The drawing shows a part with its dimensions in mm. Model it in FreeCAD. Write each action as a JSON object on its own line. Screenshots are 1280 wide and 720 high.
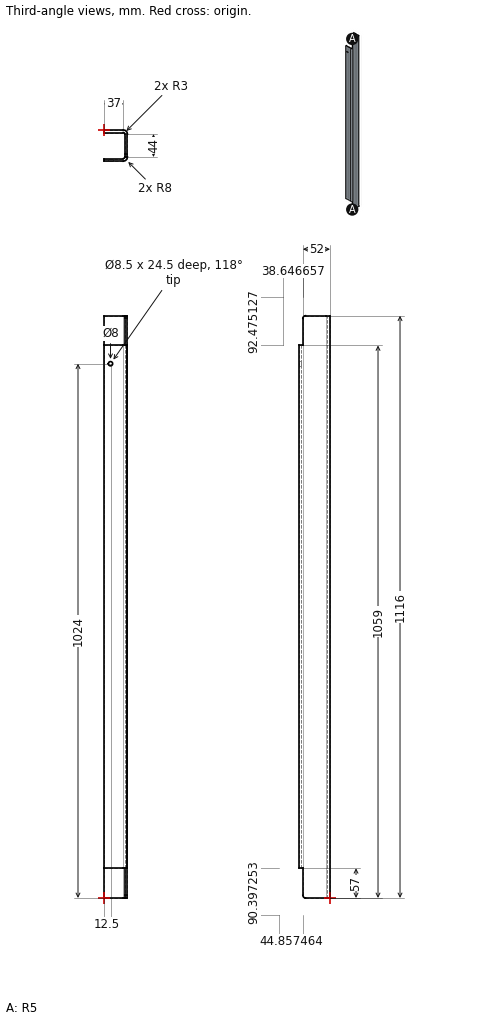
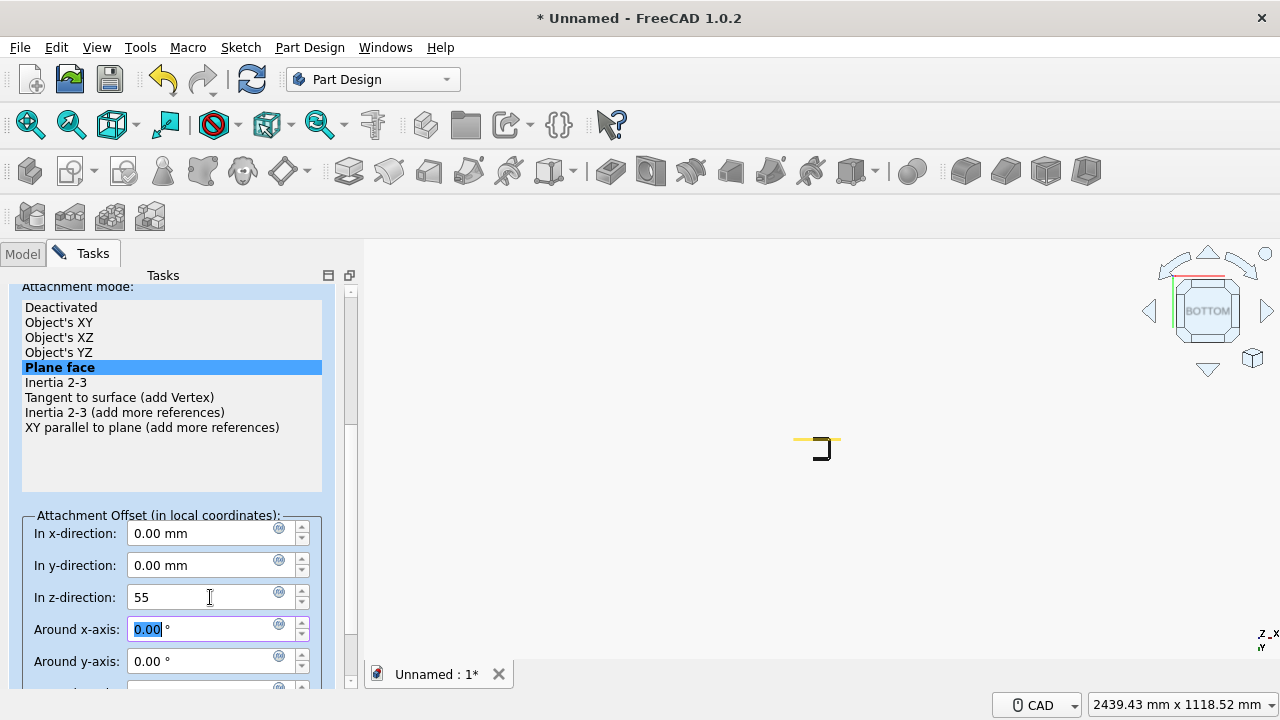
{"action": "scroll", "coordinate": [351, 486], "scroll_direction": "up", "scroll_amount": 5}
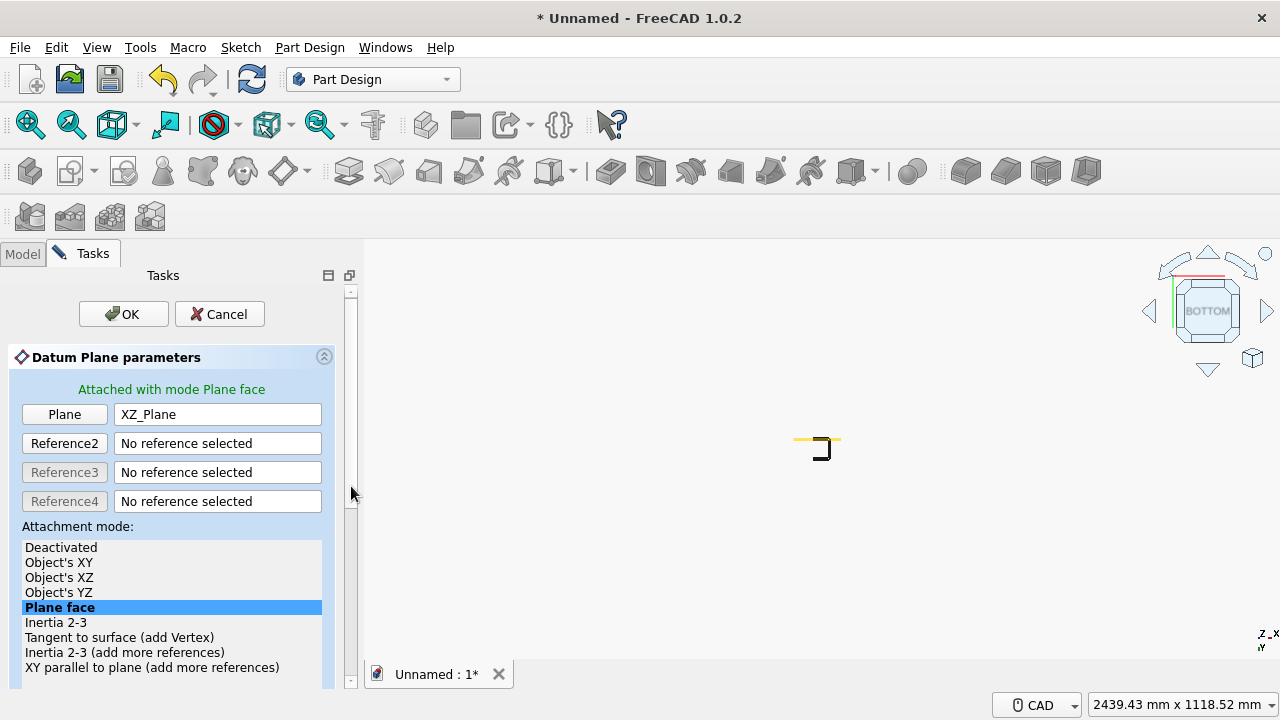
{"action": "left_click", "coordinate": [124, 314]}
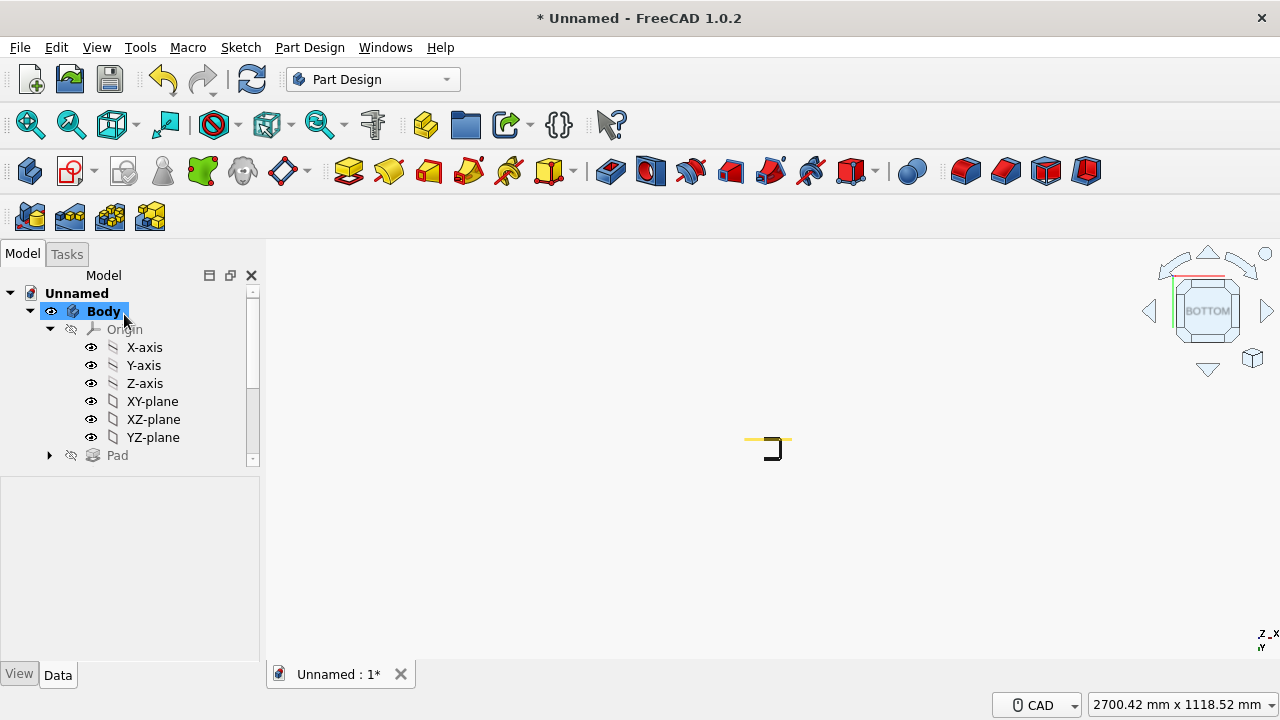
{"action": "scroll", "coordinate": [100, 379], "scroll_direction": "down", "scroll_amount": 3}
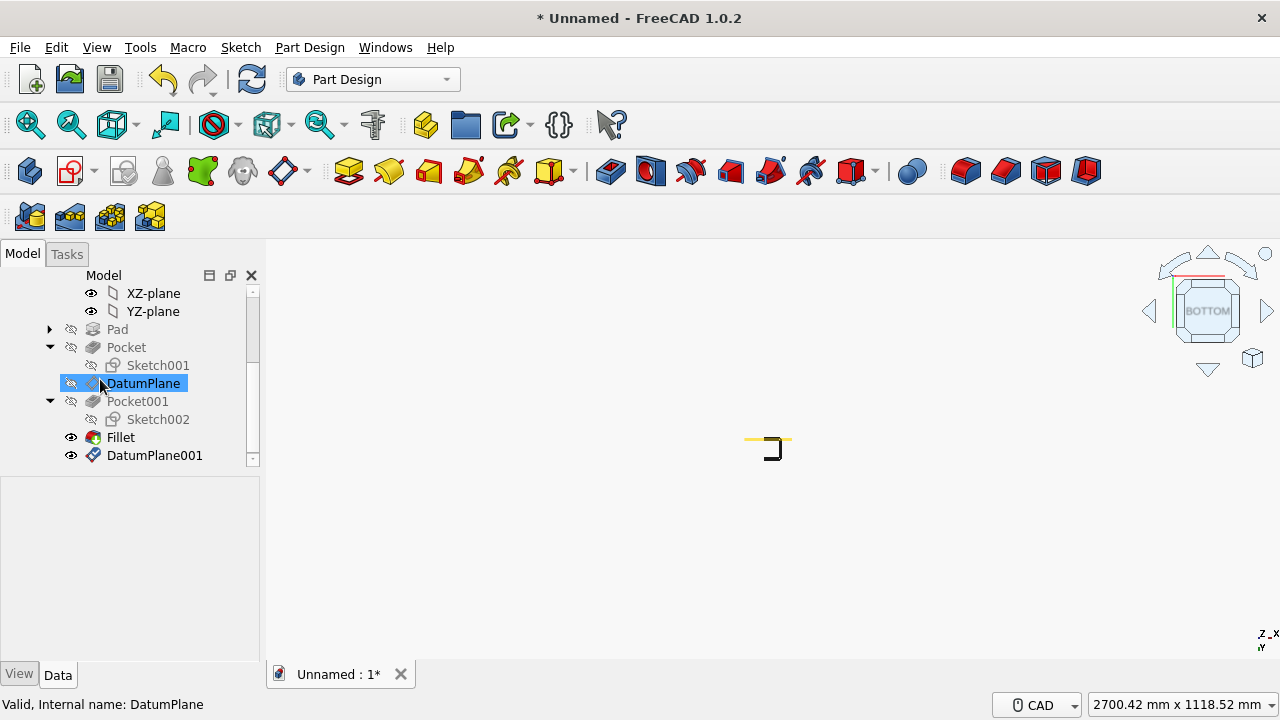
{"action": "left_click", "coordinate": [116, 455]}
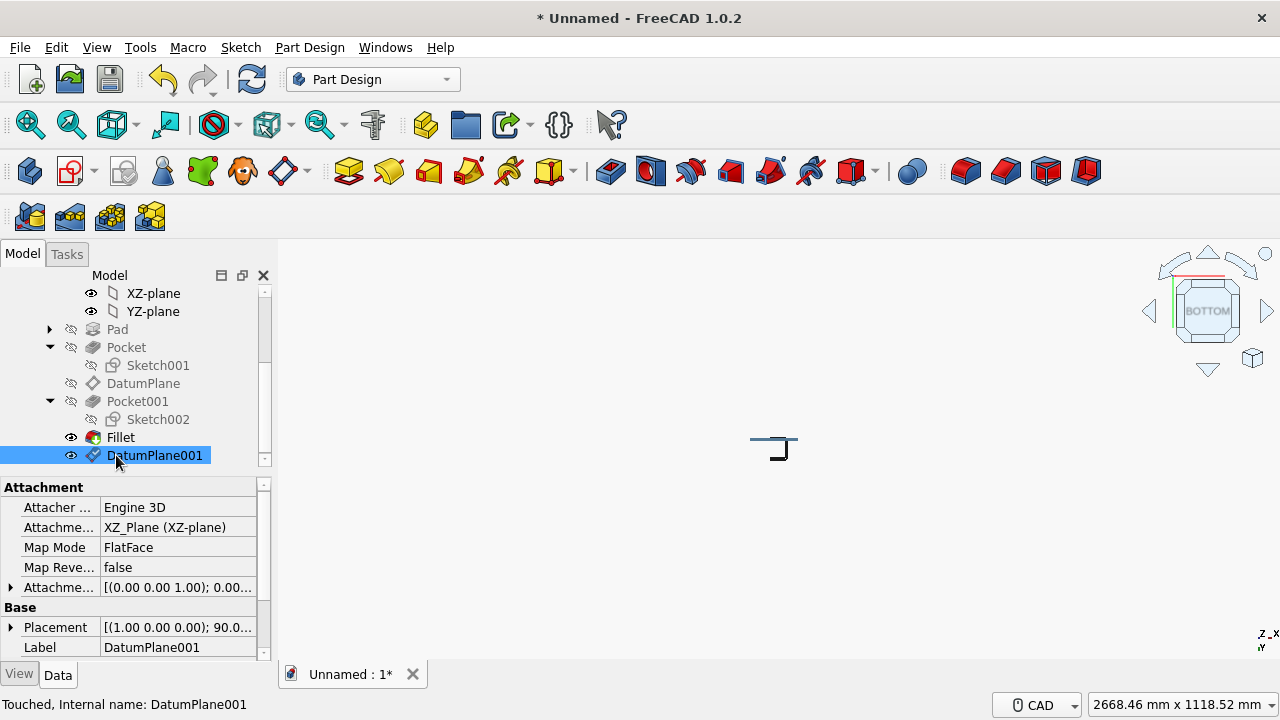
{"action": "left_click", "coordinate": [70, 172]}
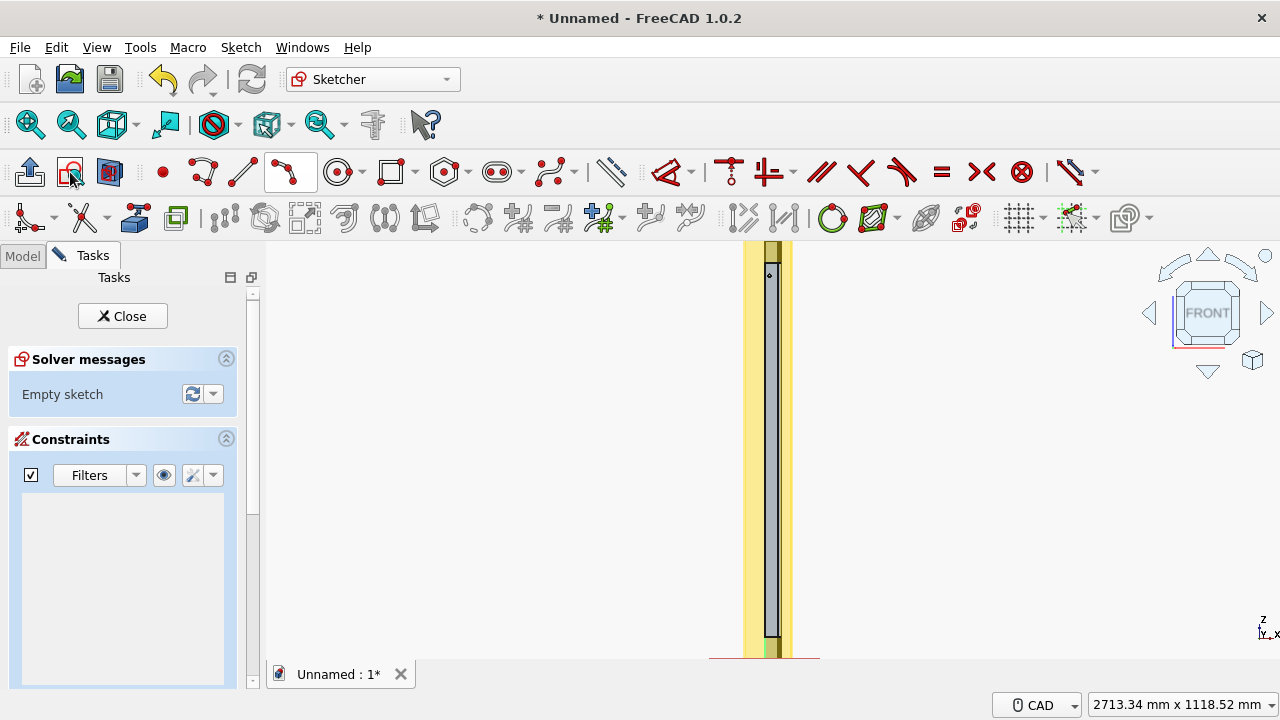
{"action": "left_click", "coordinate": [110, 172]}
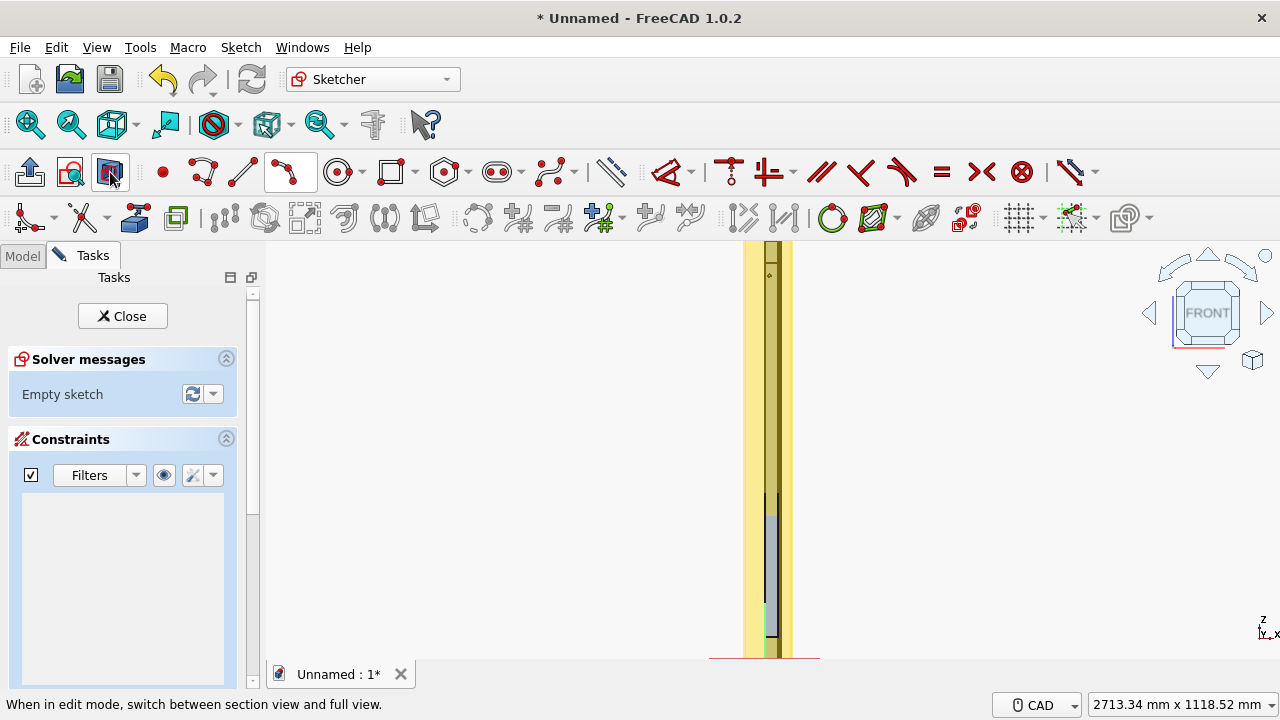
{"action": "scroll", "coordinate": [773, 269], "scroll_direction": "up", "scroll_amount": 15}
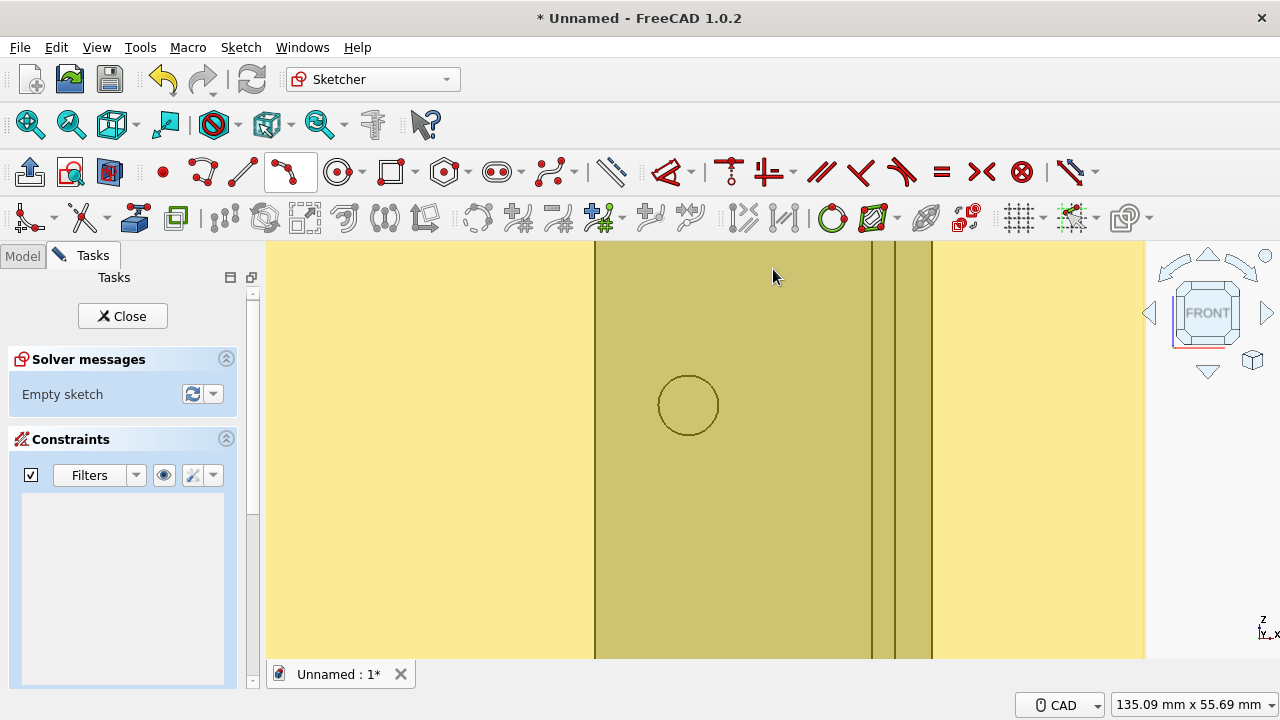
{"action": "scroll", "coordinate": [683, 391], "scroll_direction": "up", "scroll_amount": 7}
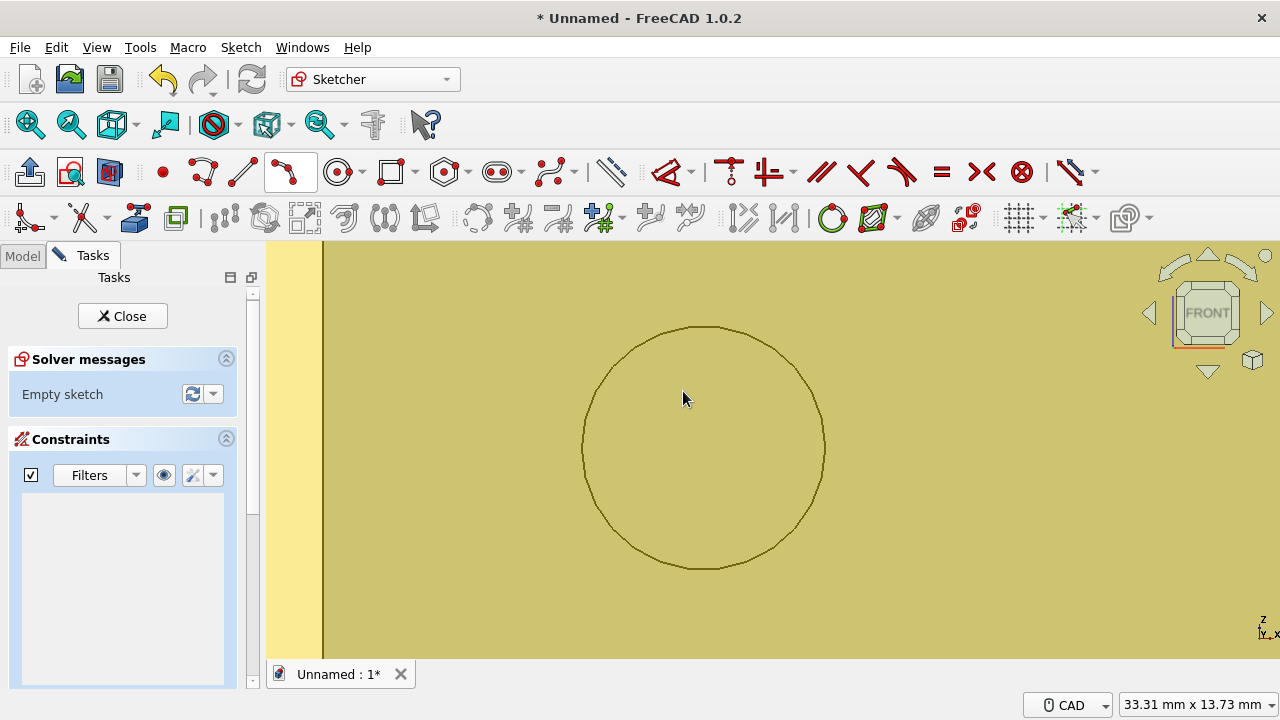
{"action": "key", "text": "g c"}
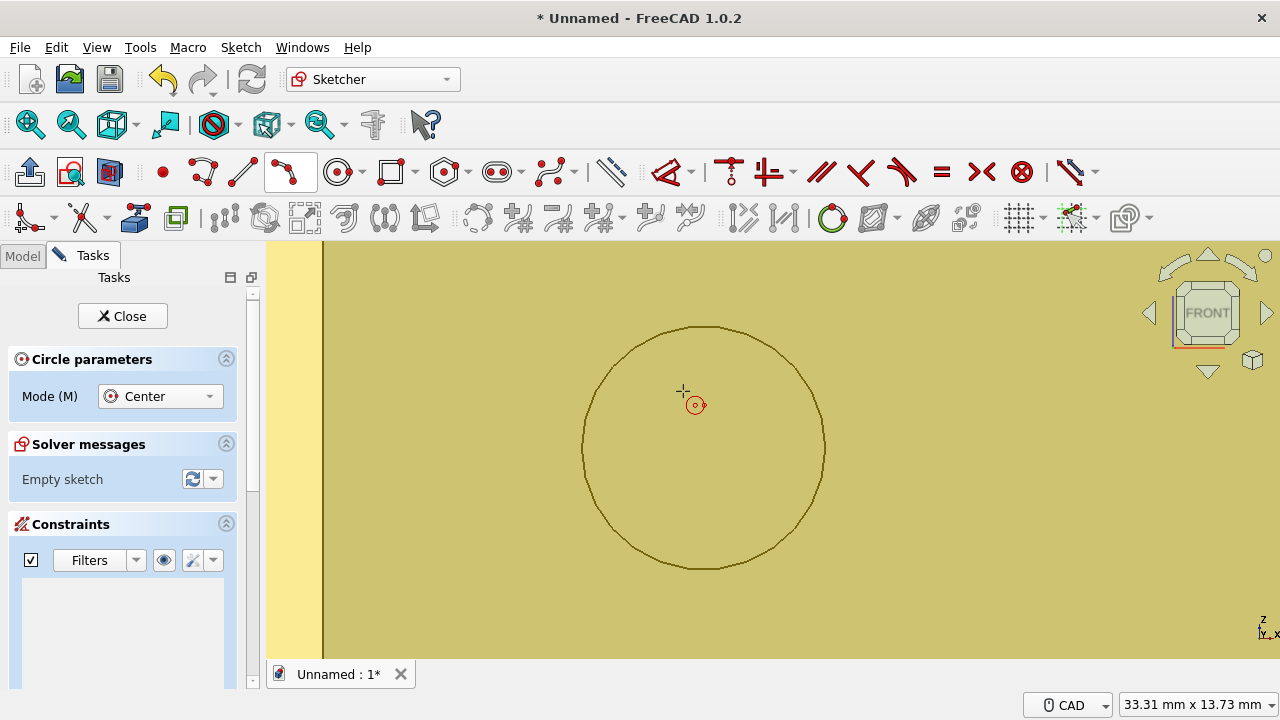
{"action": "left_click", "coordinate": [704, 448]}
{"action": "mouse_move", "coordinate": [795, 357]}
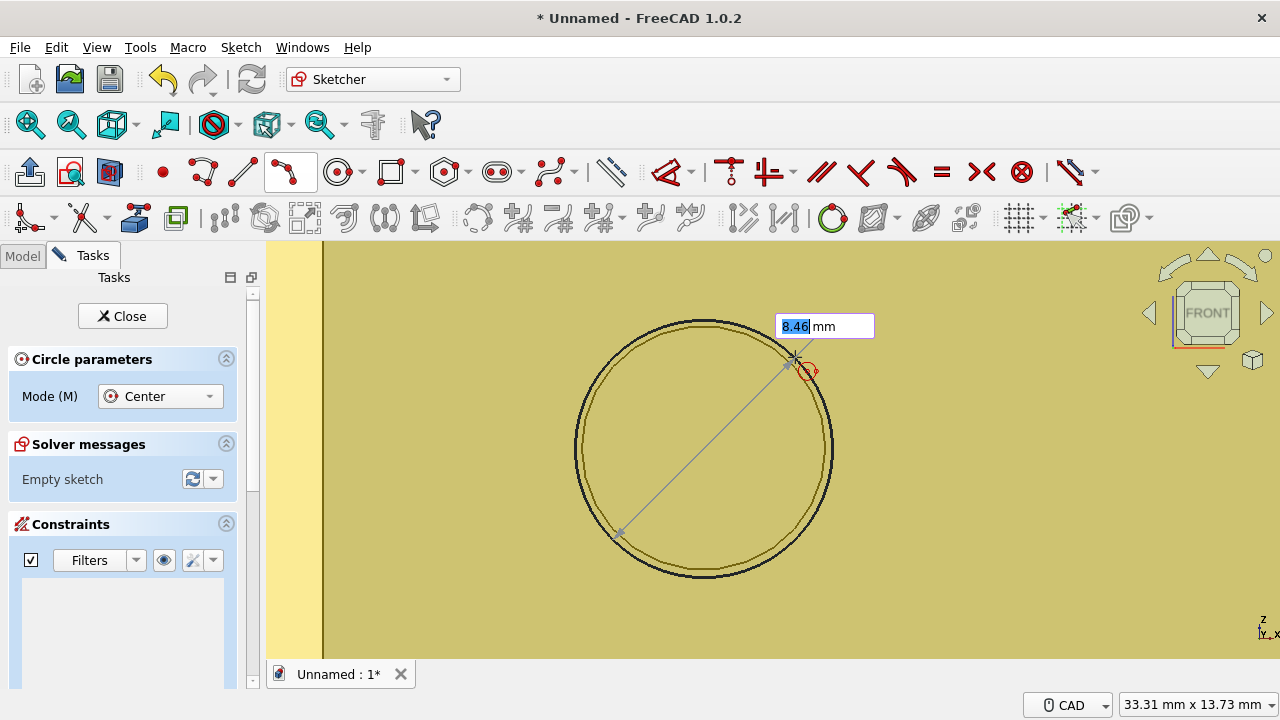
{"action": "type", "text": "8.5"}
{"action": "key", "text": "Return"}
{"action": "key", "text": "Escape"}